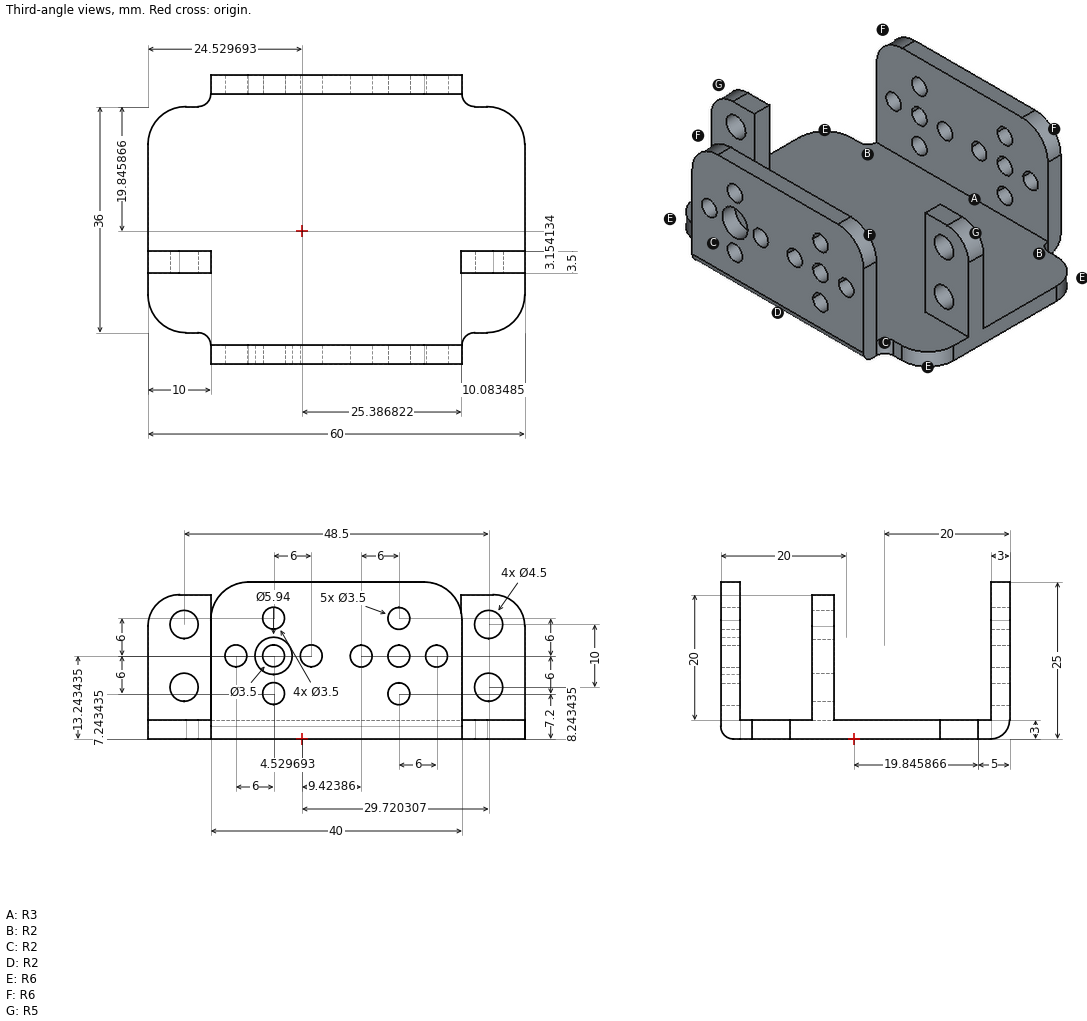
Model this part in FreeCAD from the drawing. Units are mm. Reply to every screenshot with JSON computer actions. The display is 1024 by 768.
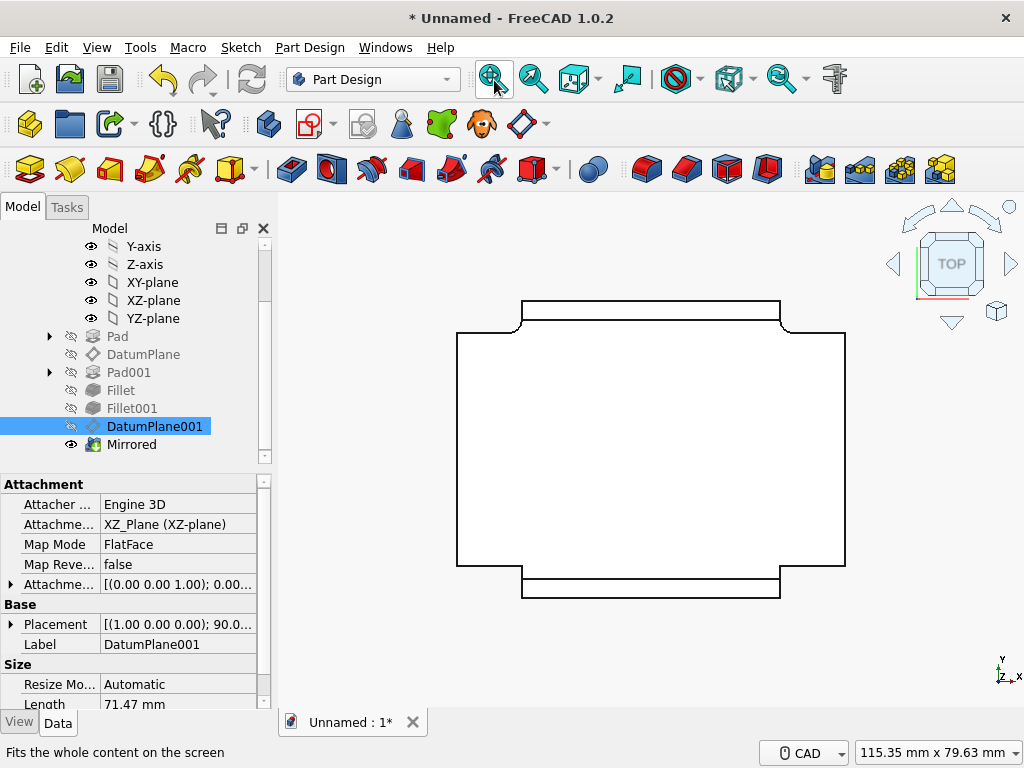
{"action": "scroll", "coordinate": [780, 565], "scroll_direction": "up", "scroll_amount": 4}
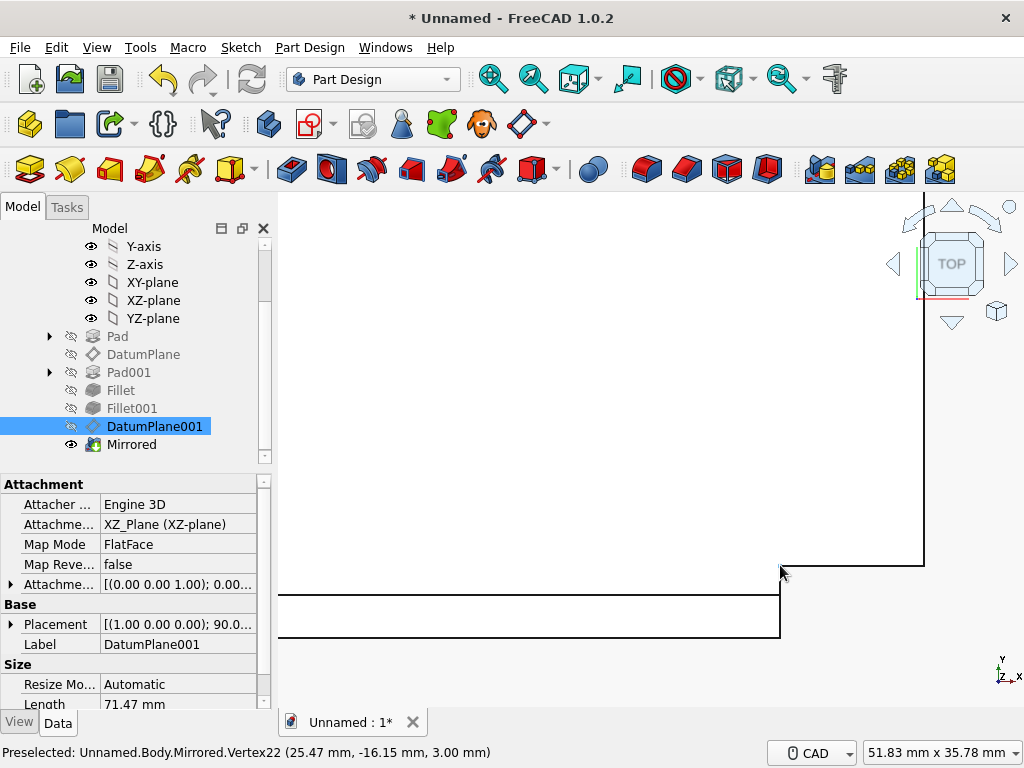
{"action": "left_click", "coordinate": [494, 80]}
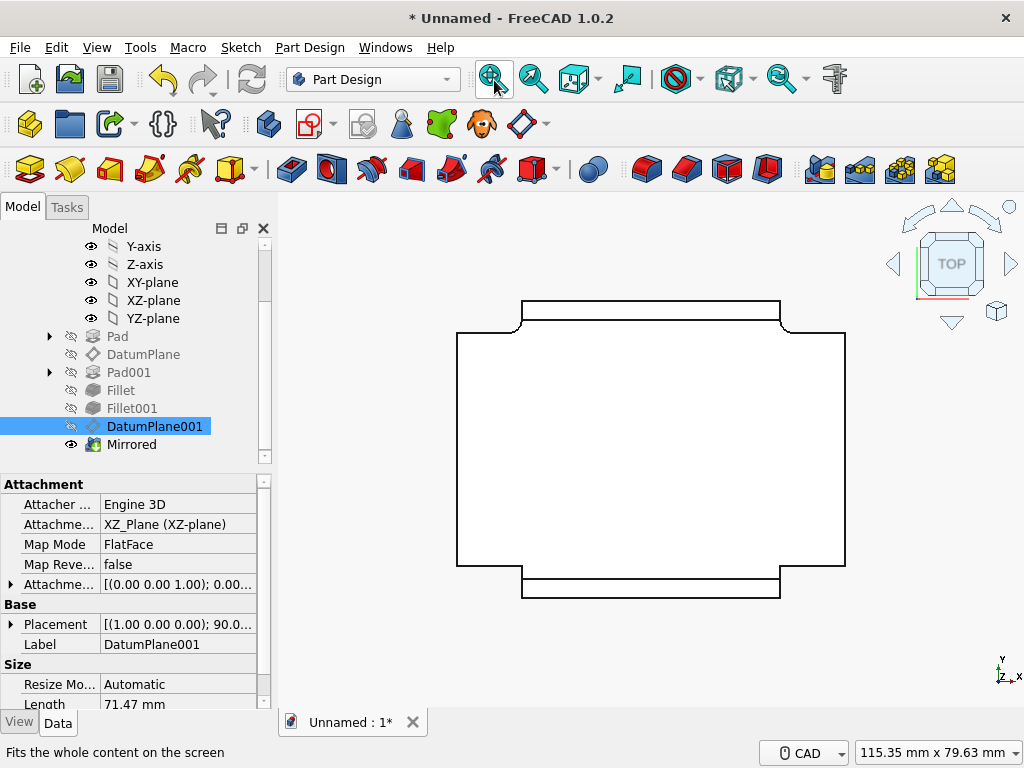
{"action": "key", "text": "0"}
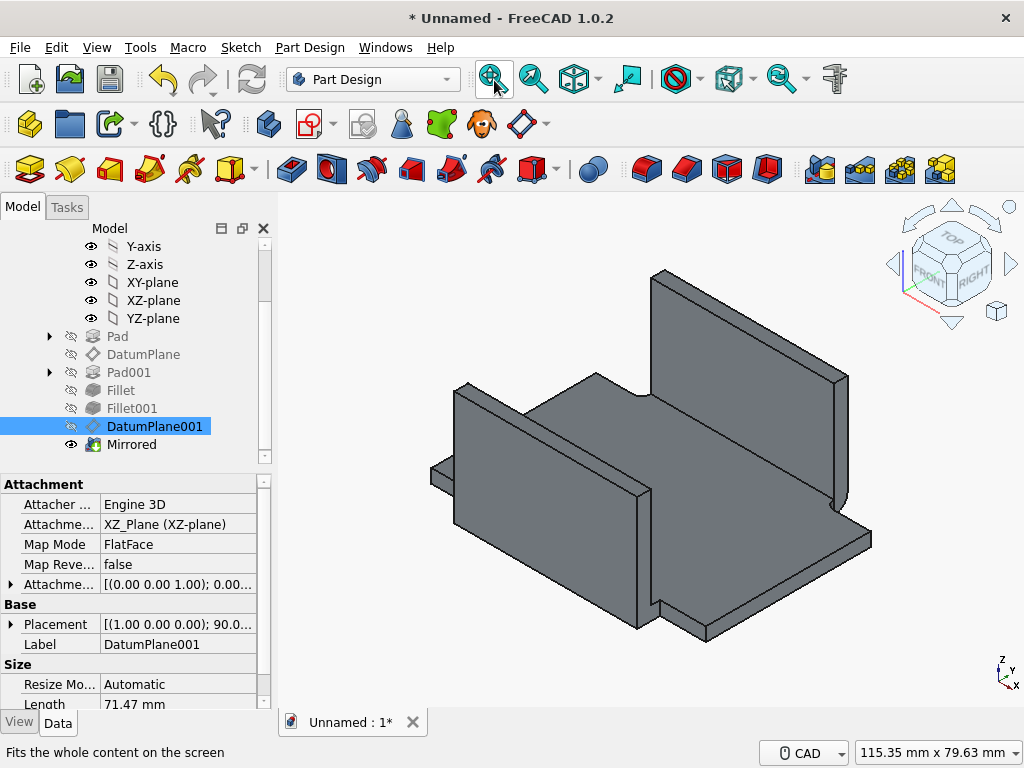
{"action": "scroll", "coordinate": [660, 607], "scroll_direction": "up", "scroll_amount": 4}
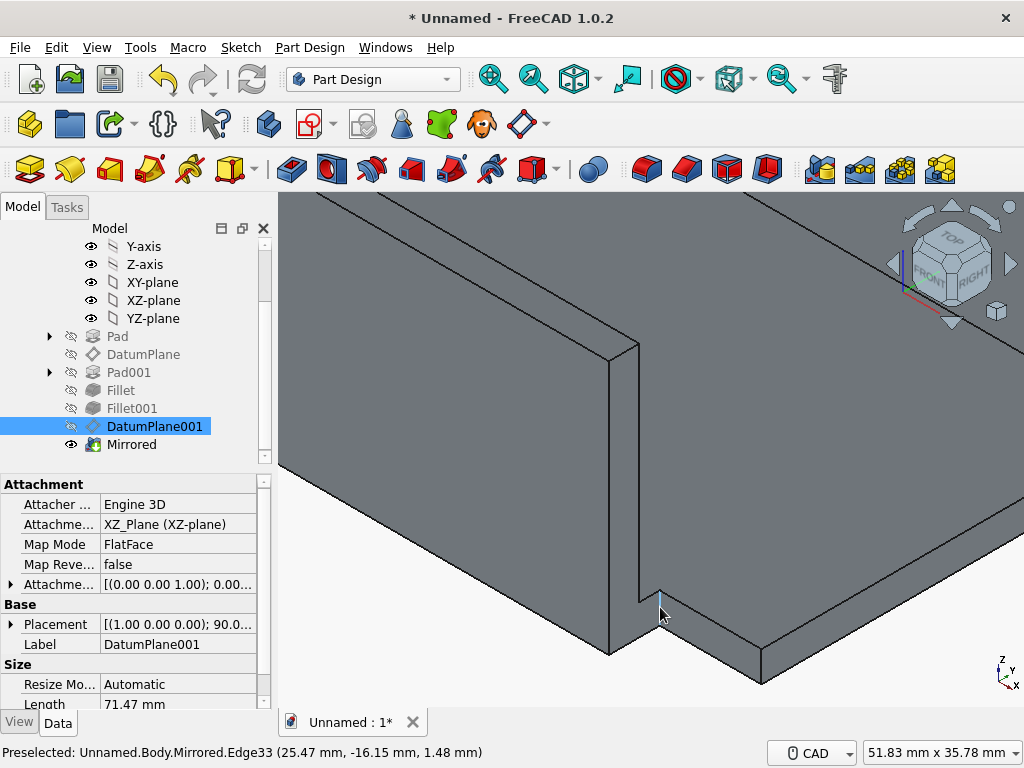
{"action": "left_click", "coordinate": [494, 80]}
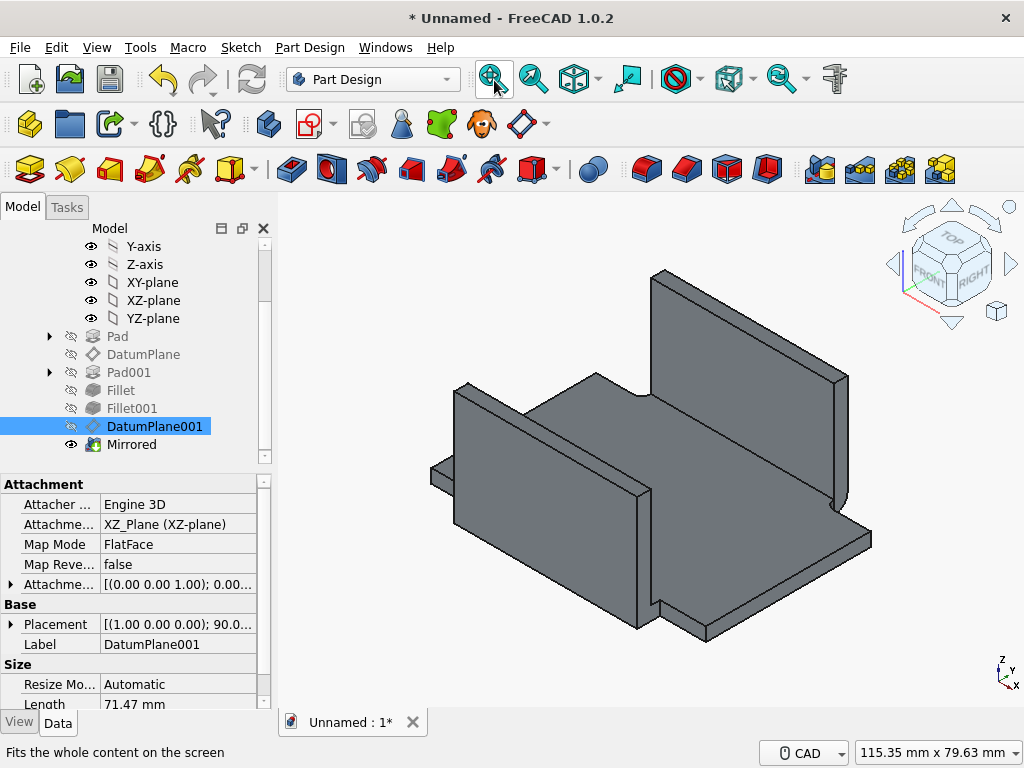
{"action": "key", "text": "1"}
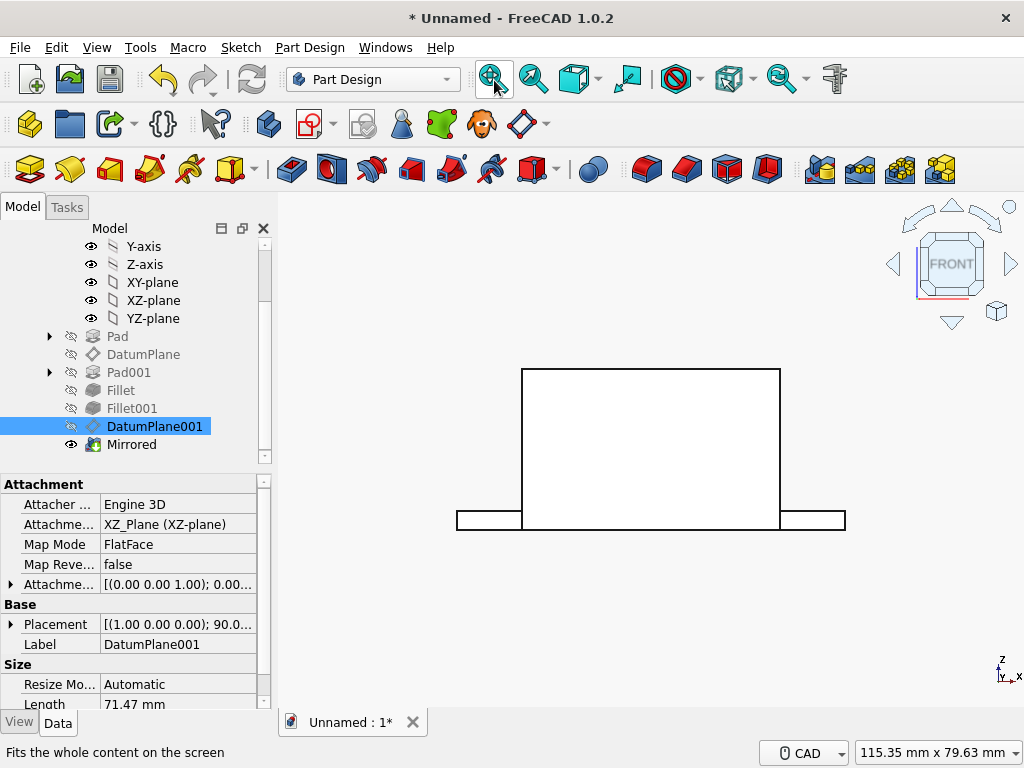
{"action": "scroll", "coordinate": [780, 520], "scroll_direction": "up", "scroll_amount": 4}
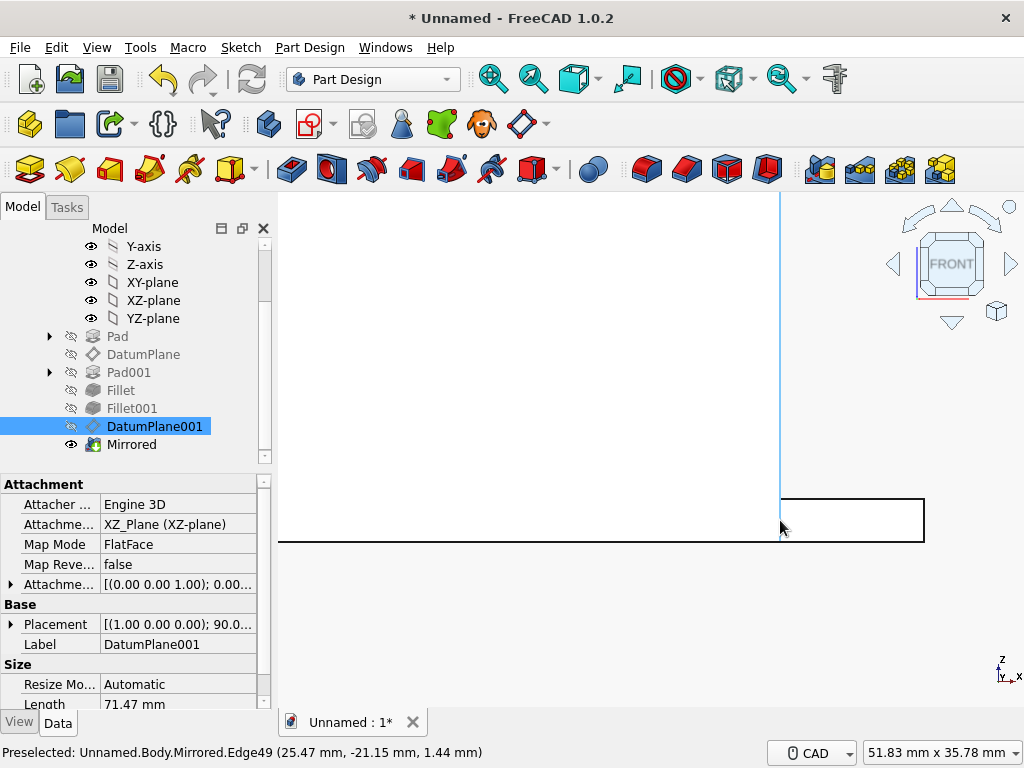
{"action": "left_click", "coordinate": [494, 80]}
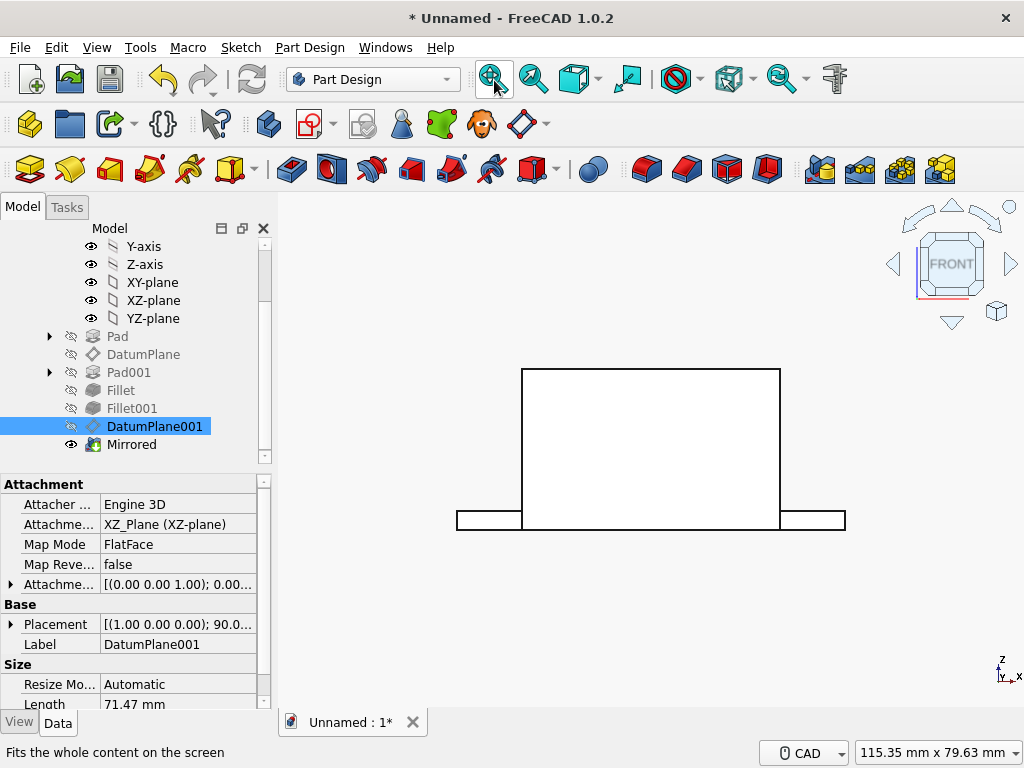
{"action": "key", "text": "3"}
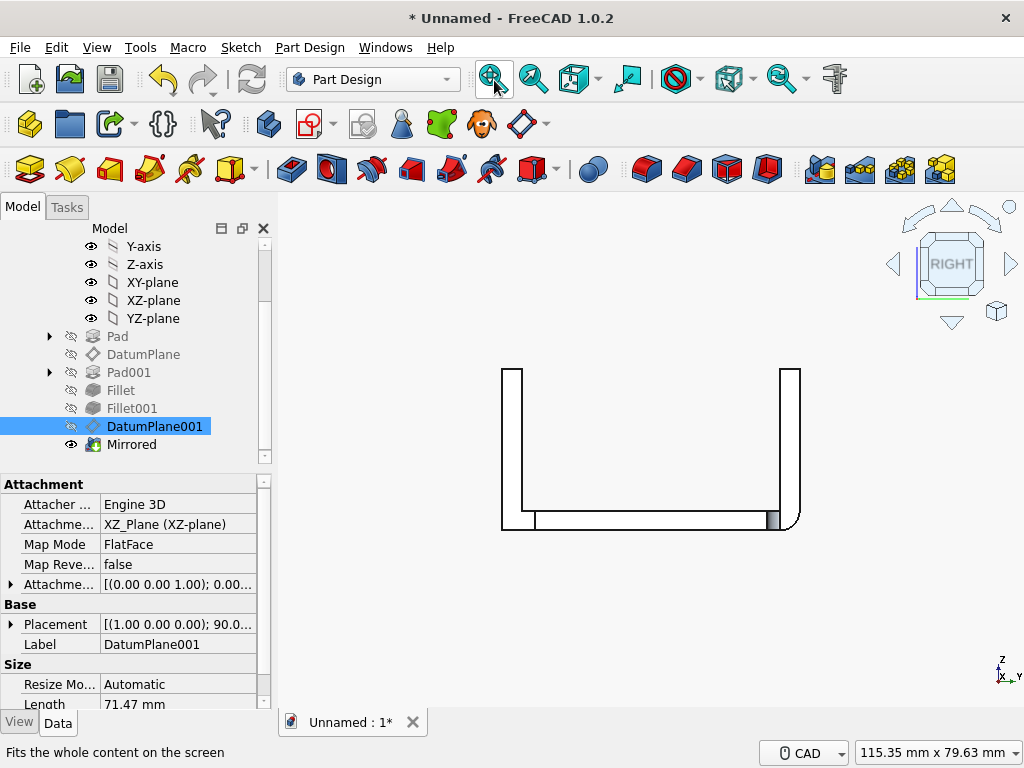
{"action": "left_click", "coordinate": [494, 80]}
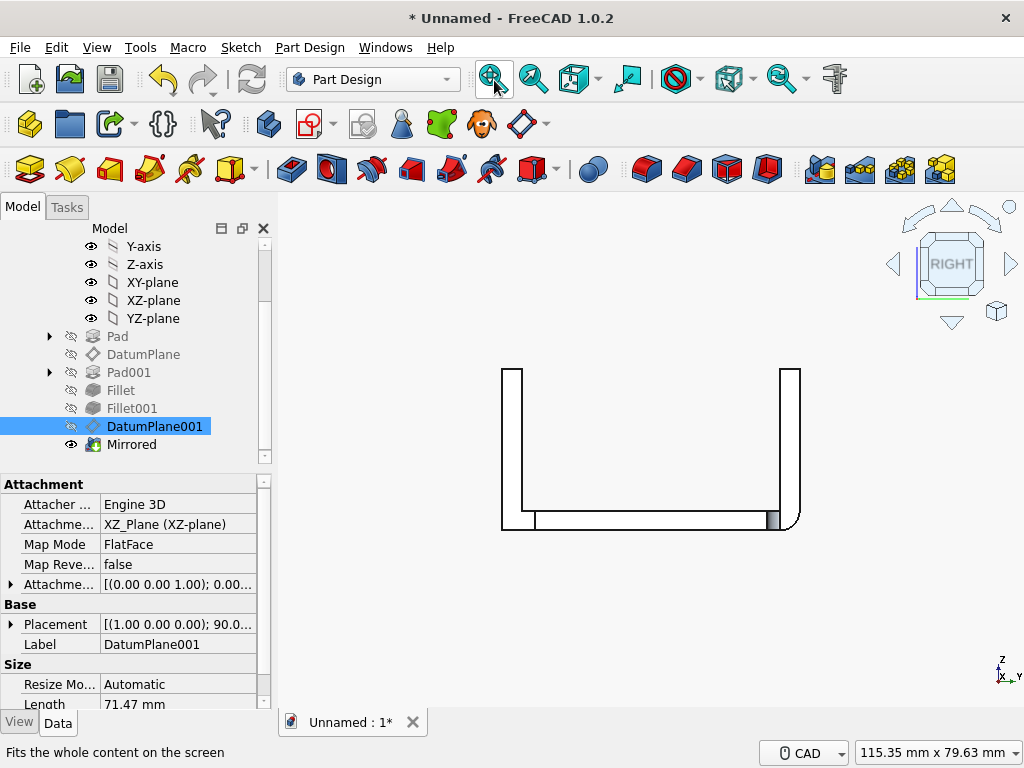
{"action": "scroll", "coordinate": [535, 520], "scroll_direction": "up", "scroll_amount": 4}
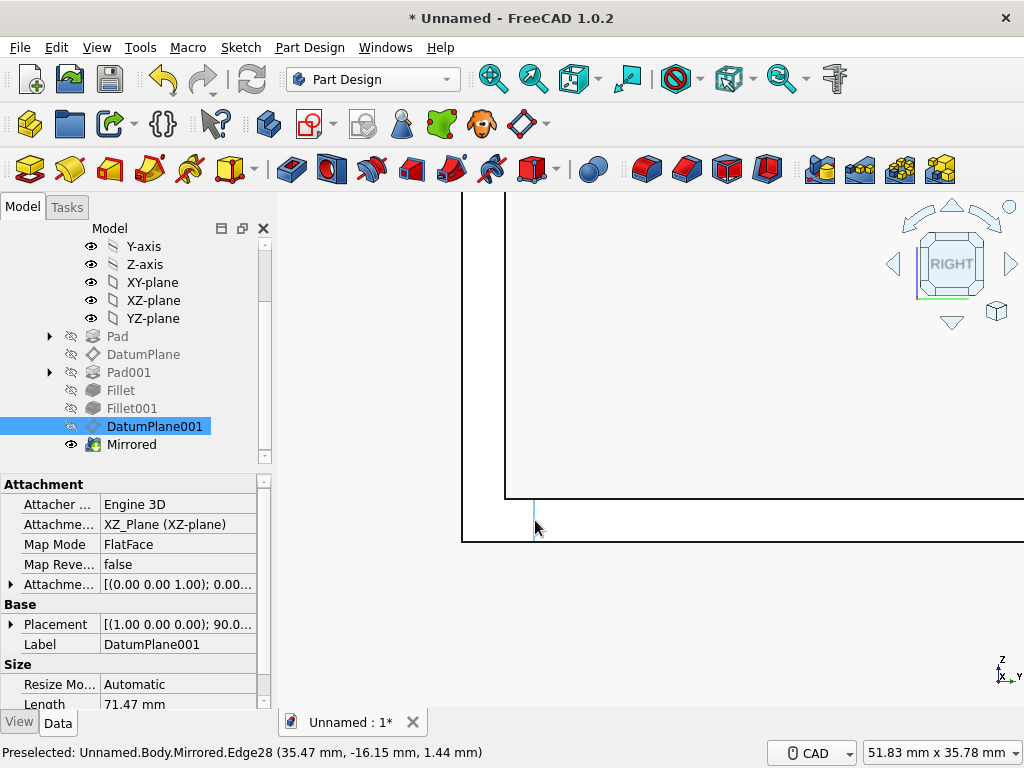
{"action": "left_click", "coordinate": [494, 80]}